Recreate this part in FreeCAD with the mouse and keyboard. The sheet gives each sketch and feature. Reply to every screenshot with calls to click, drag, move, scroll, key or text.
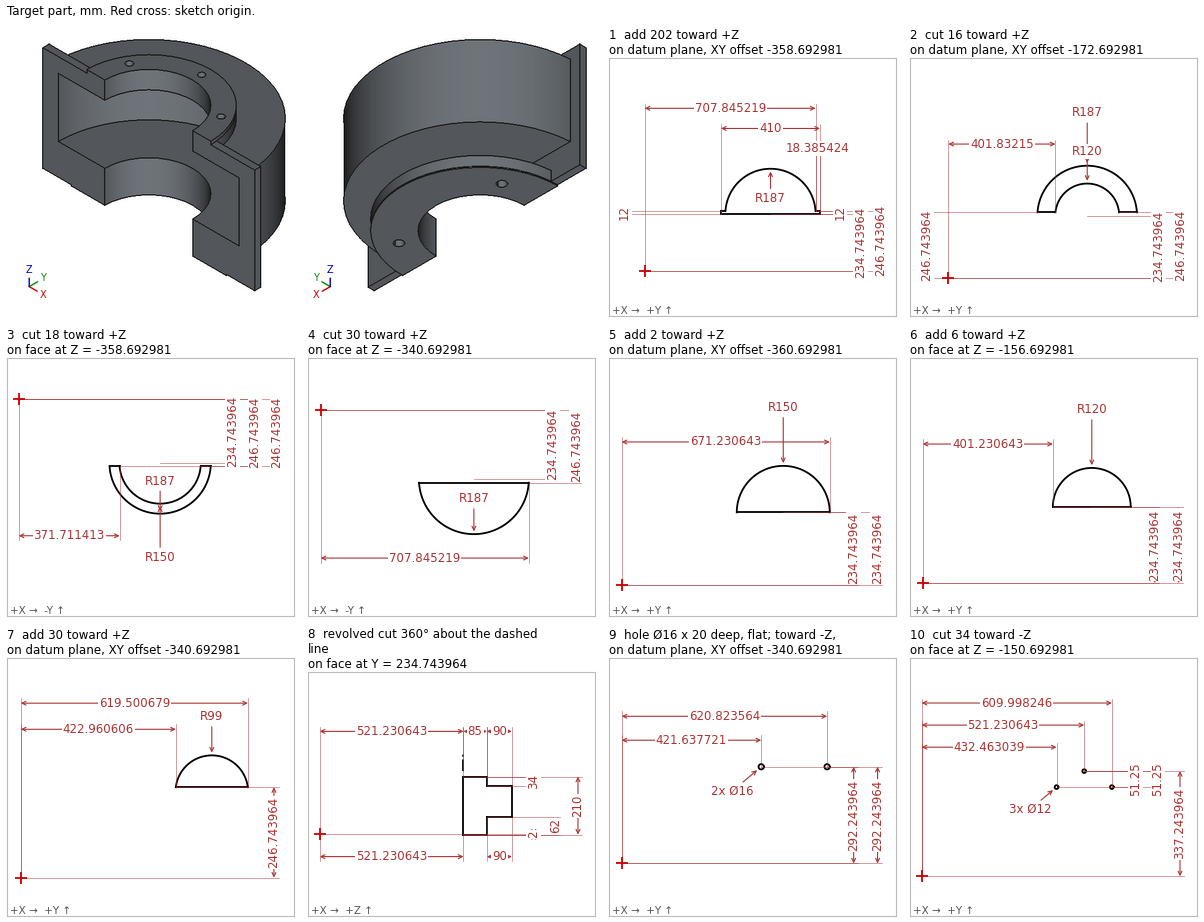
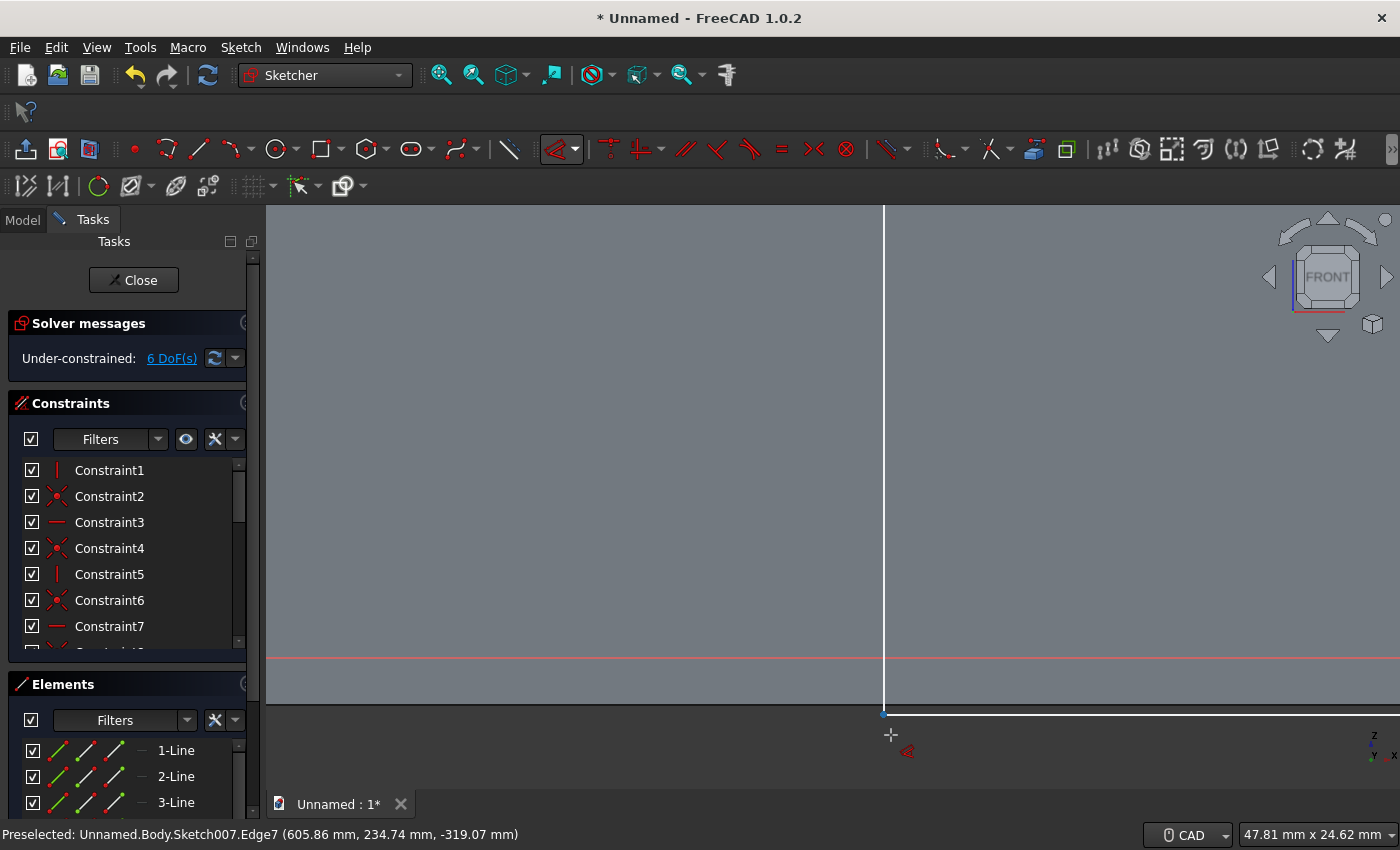
click(884, 715)
click(918, 686)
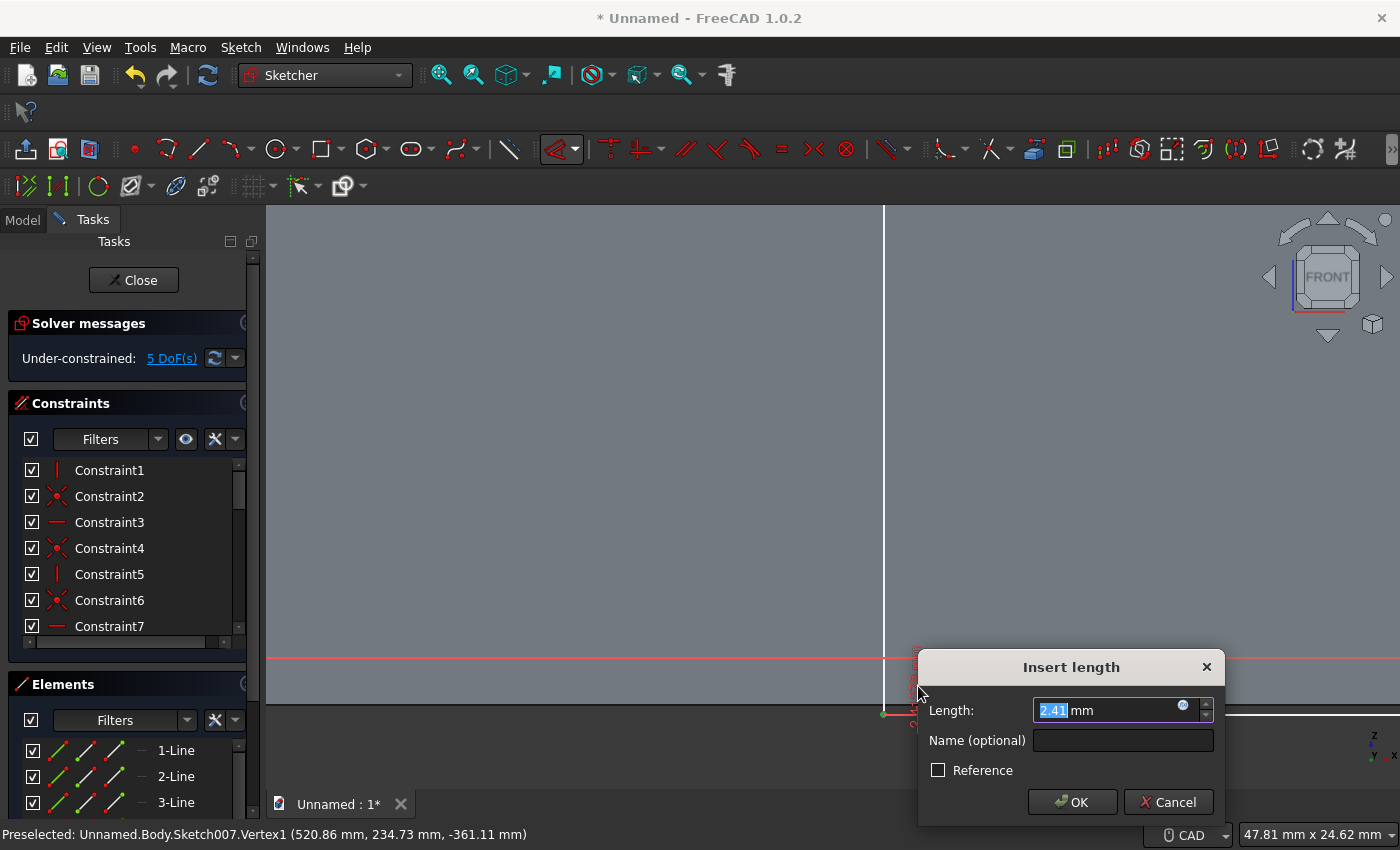
text(2)
key(Return)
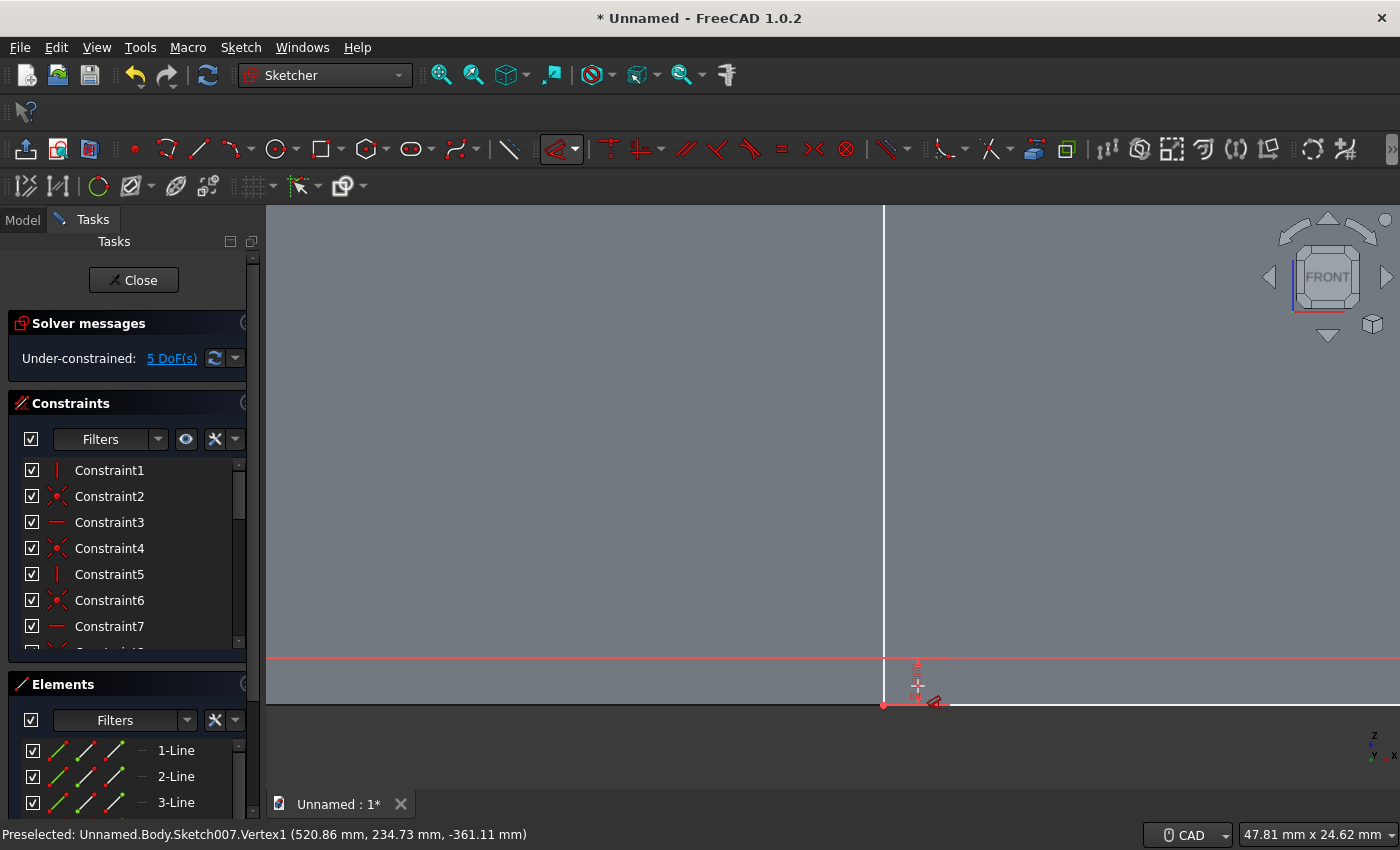
scroll(973, 669, down, 15)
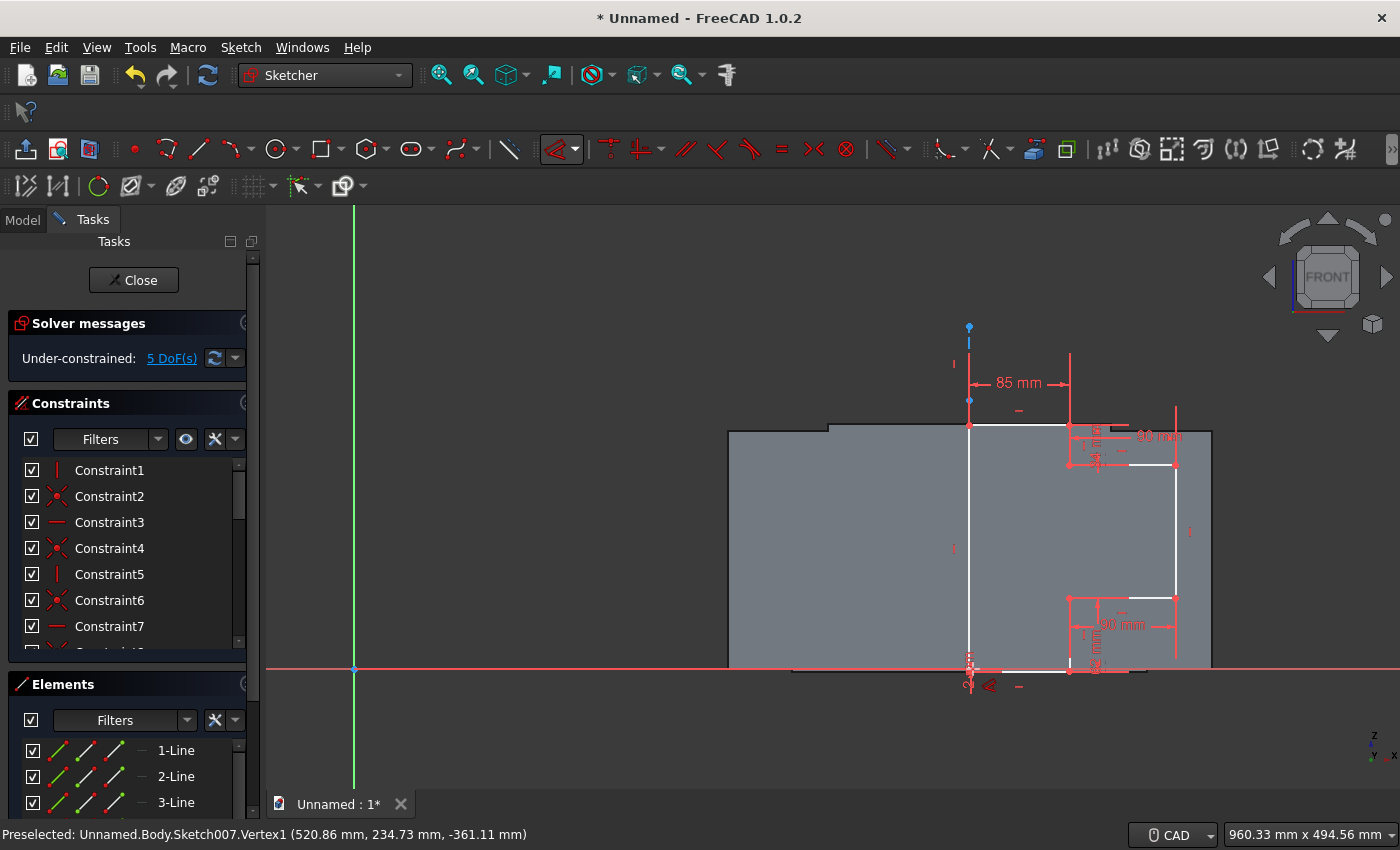
click(969, 598)
click(1003, 548)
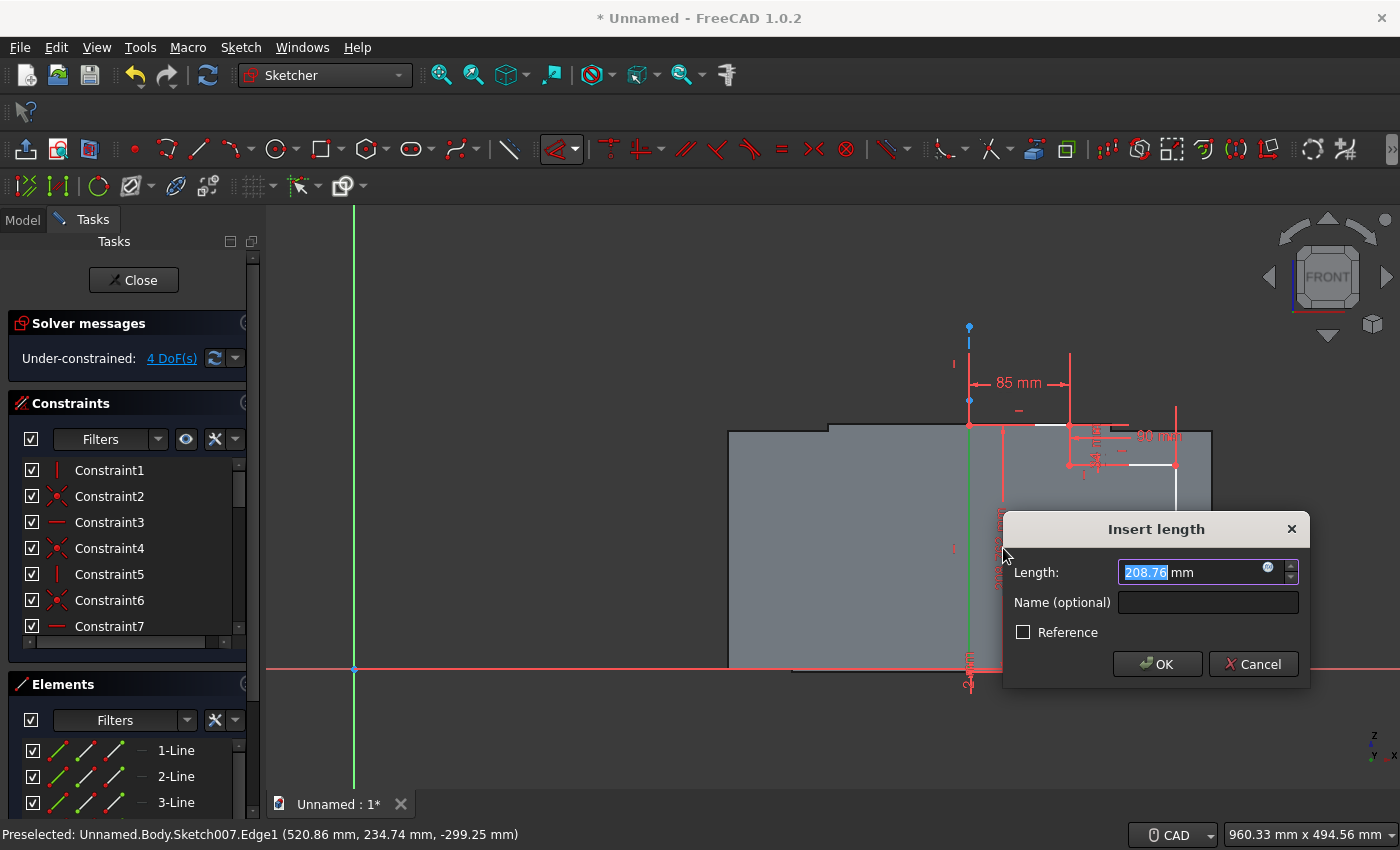
text(210)
key(Return)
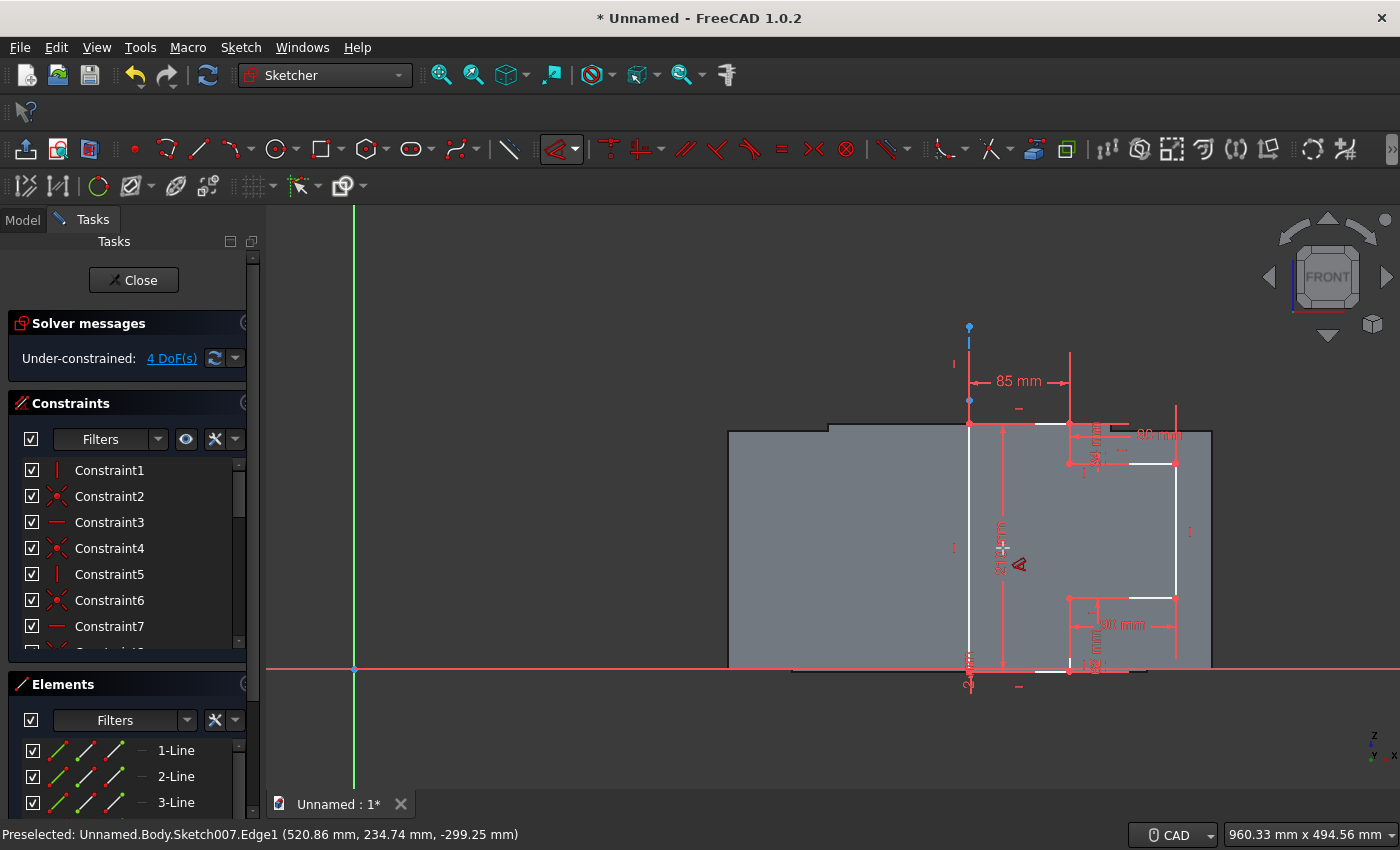
click(969, 672)
click(662, 706)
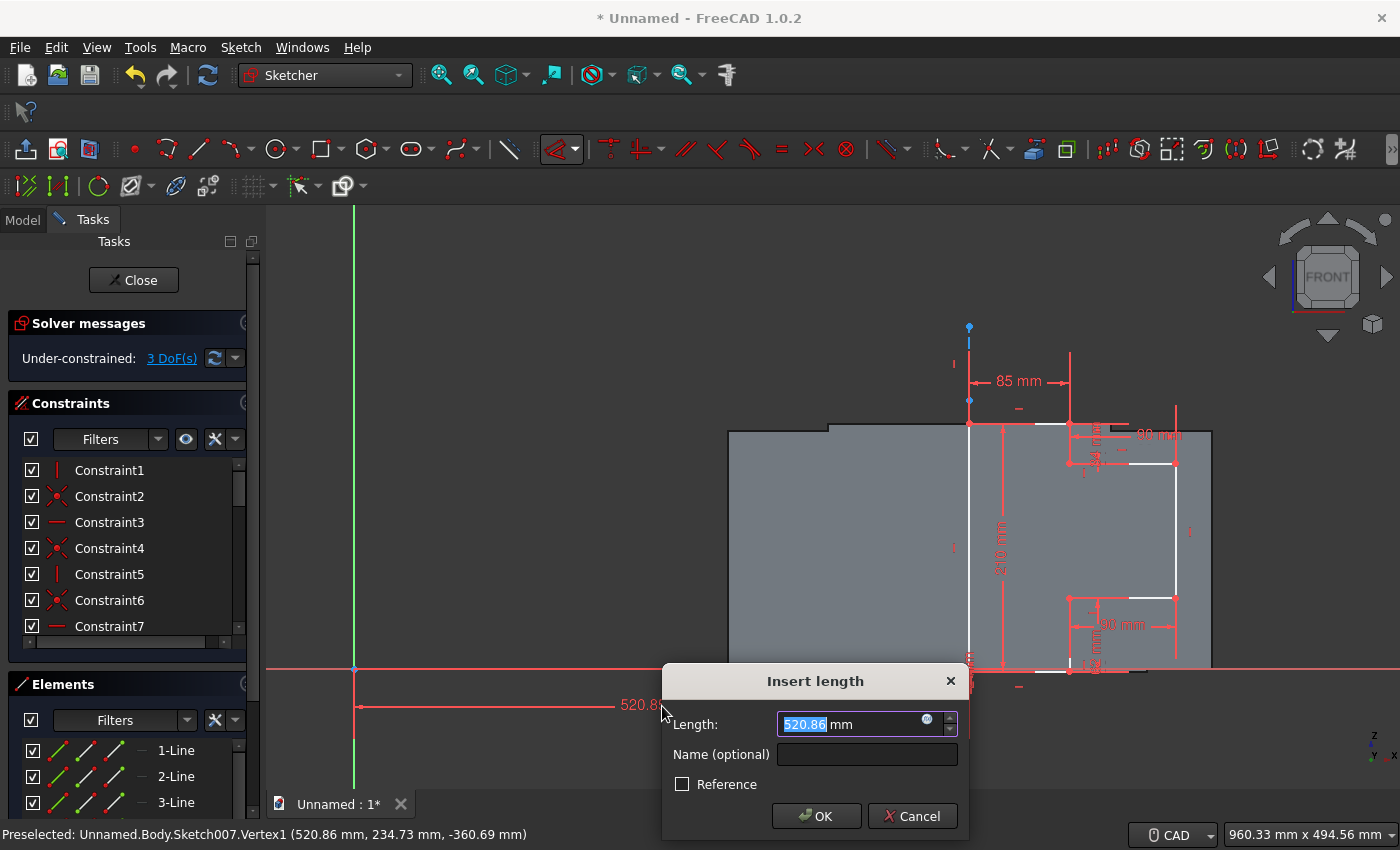
text(521.230643)
key(Return)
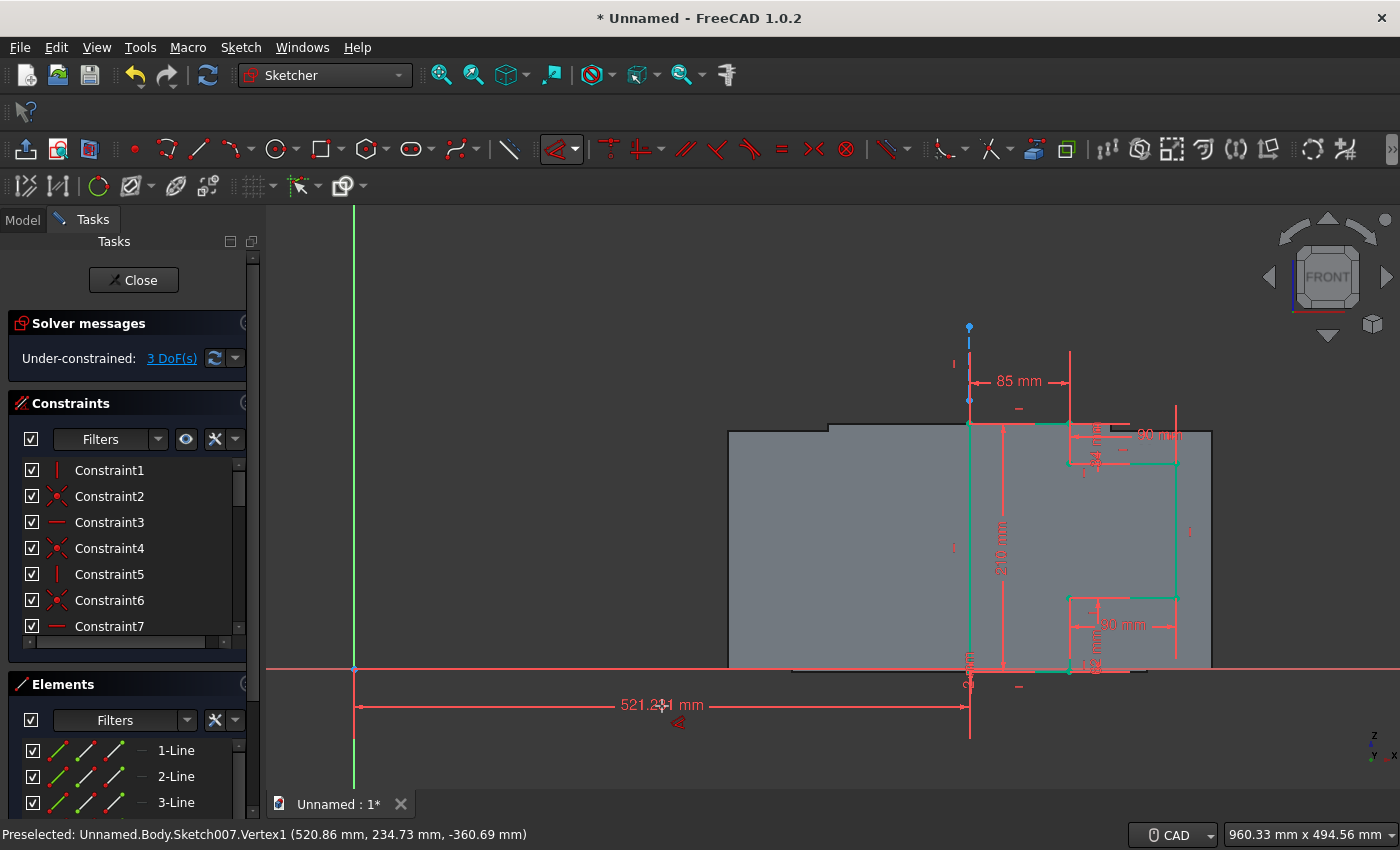
click(969, 401)
click(520, 703)